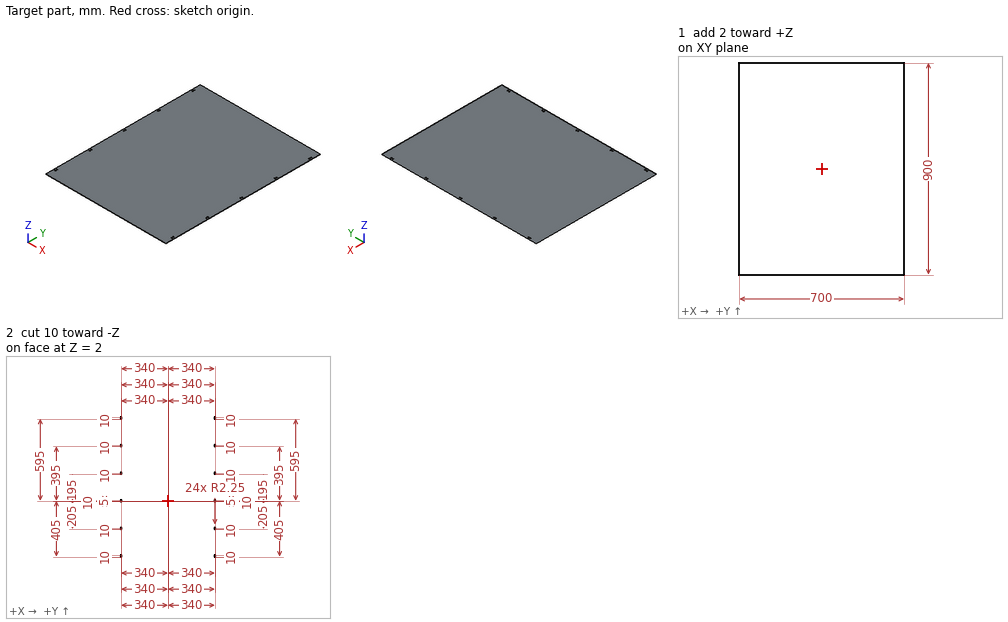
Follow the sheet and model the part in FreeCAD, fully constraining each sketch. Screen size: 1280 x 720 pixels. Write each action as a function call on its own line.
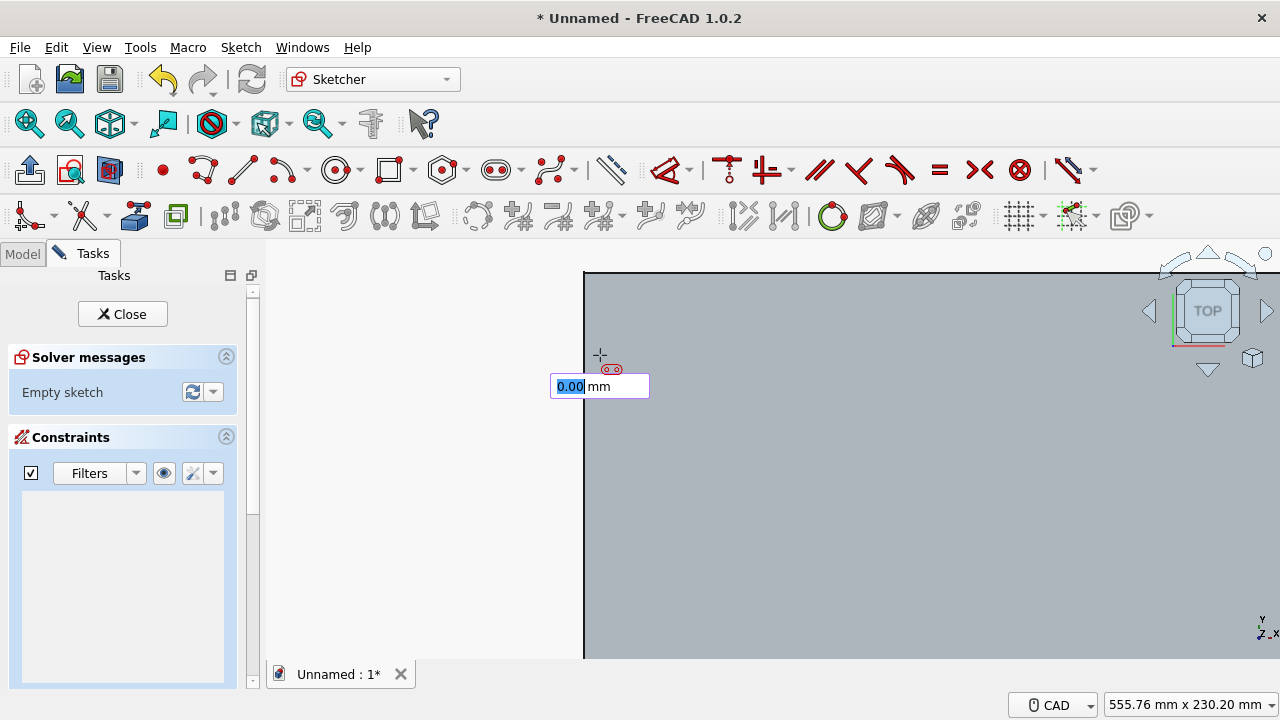
scroll(606, 364, up, 7)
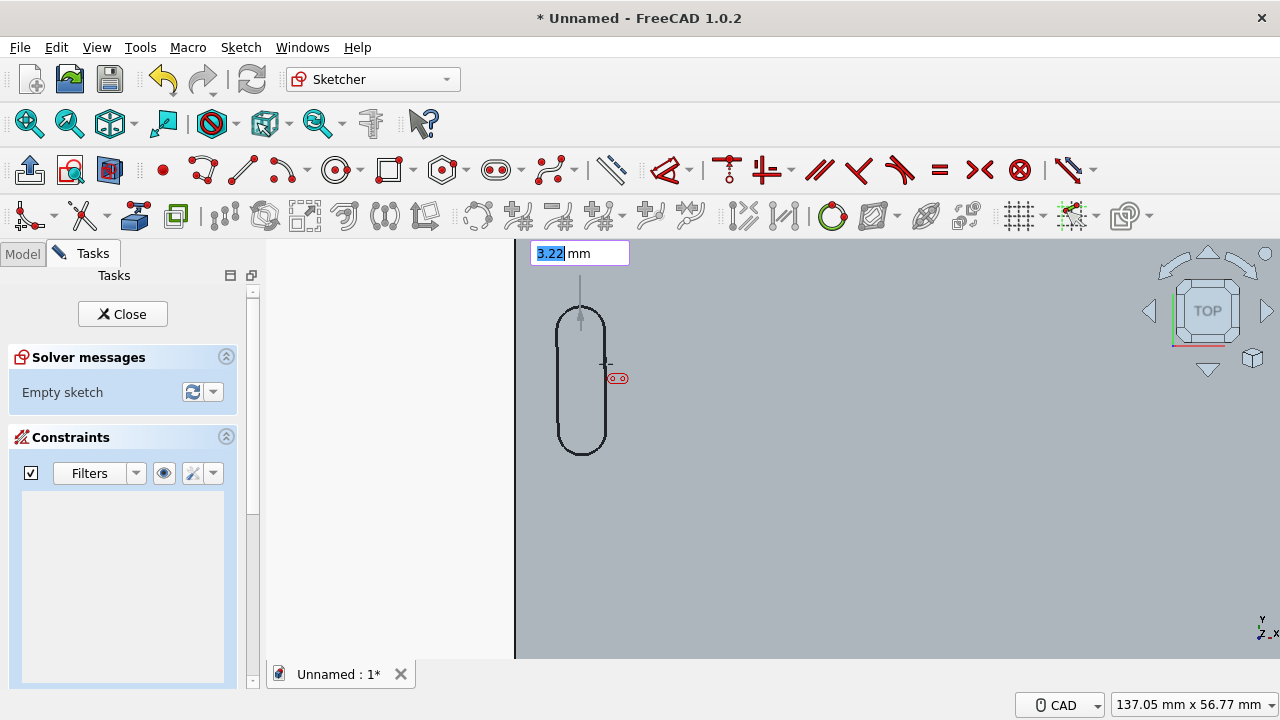
click(606, 362)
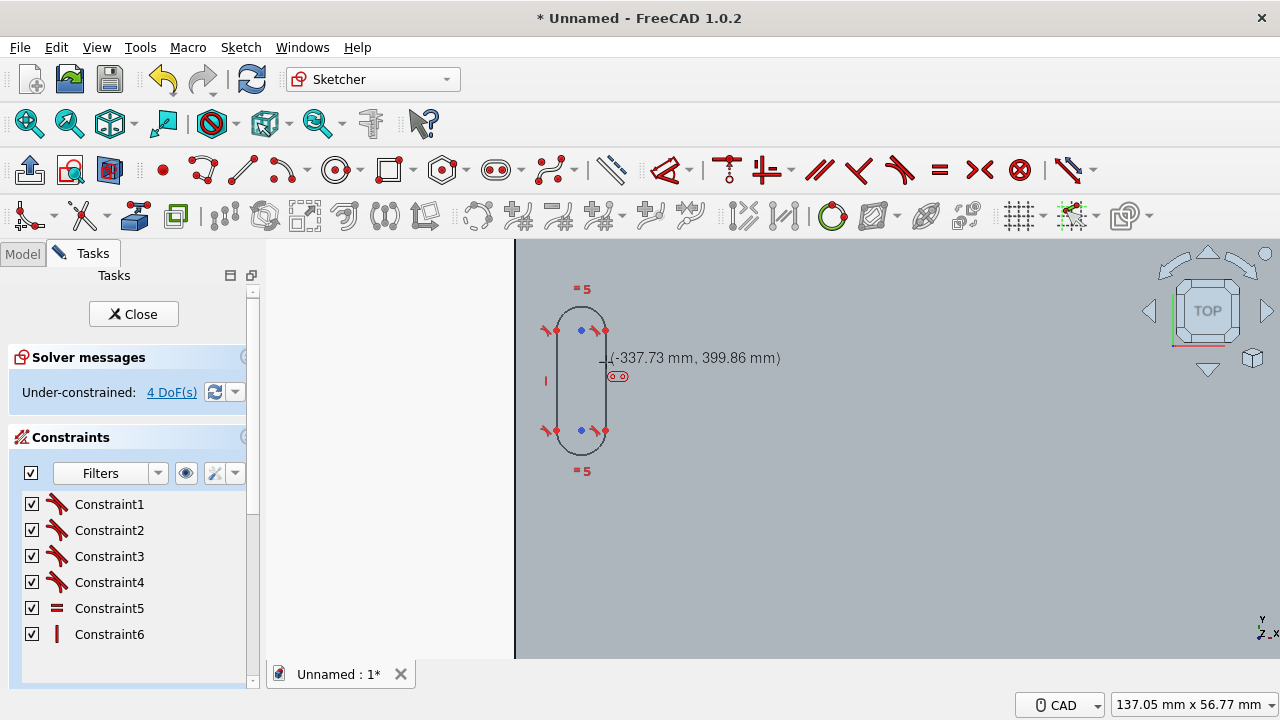
scroll(603, 358, down, 16)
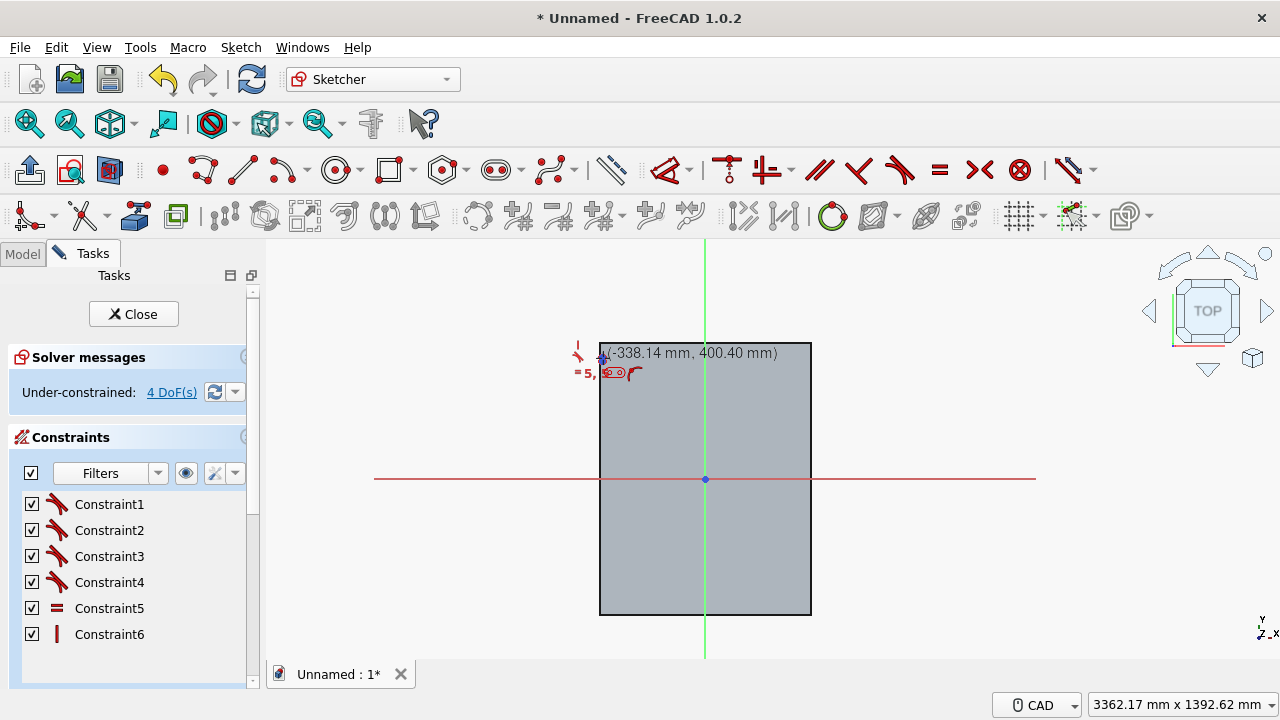
scroll(808, 360, up, 18)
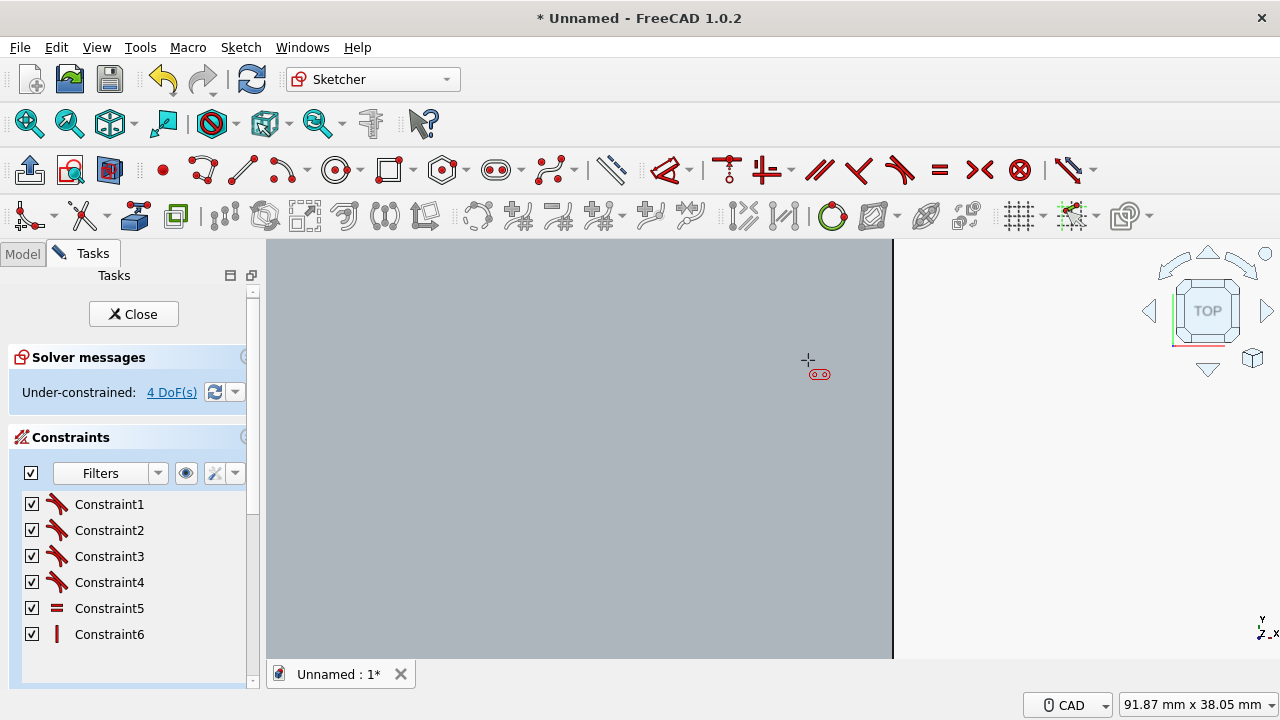
scroll(808, 360, down, 18)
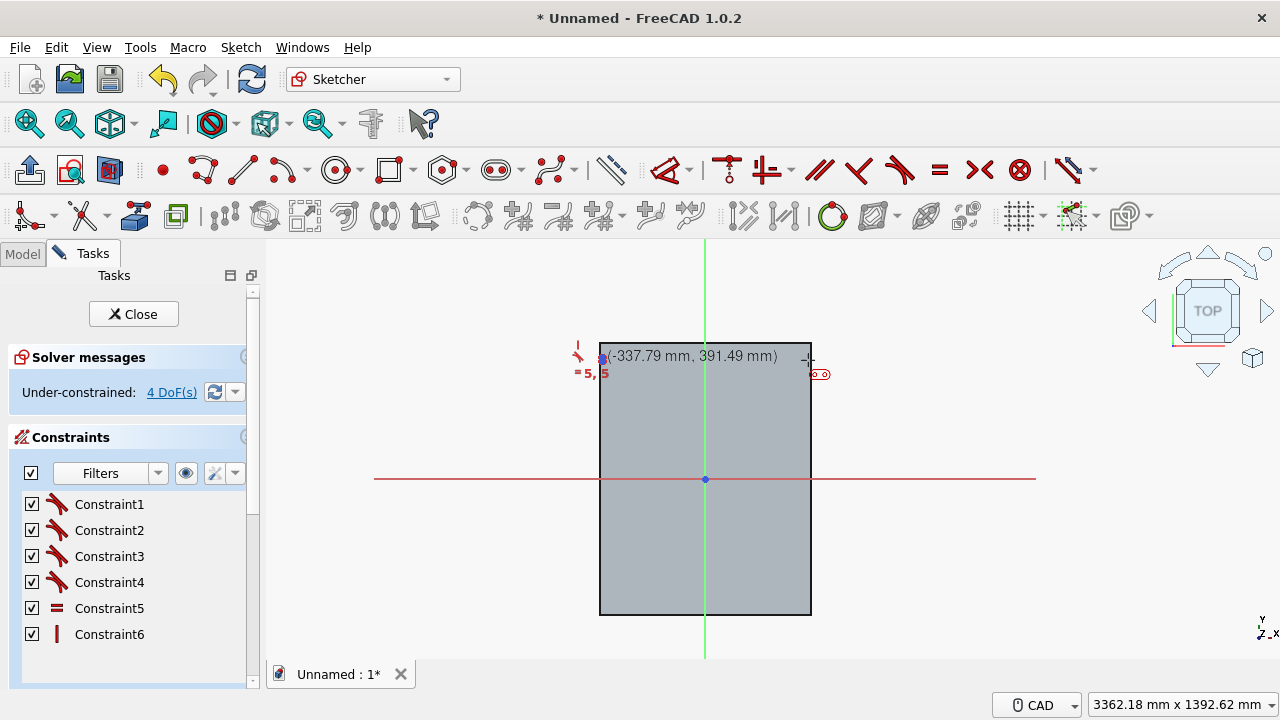
click(808, 360)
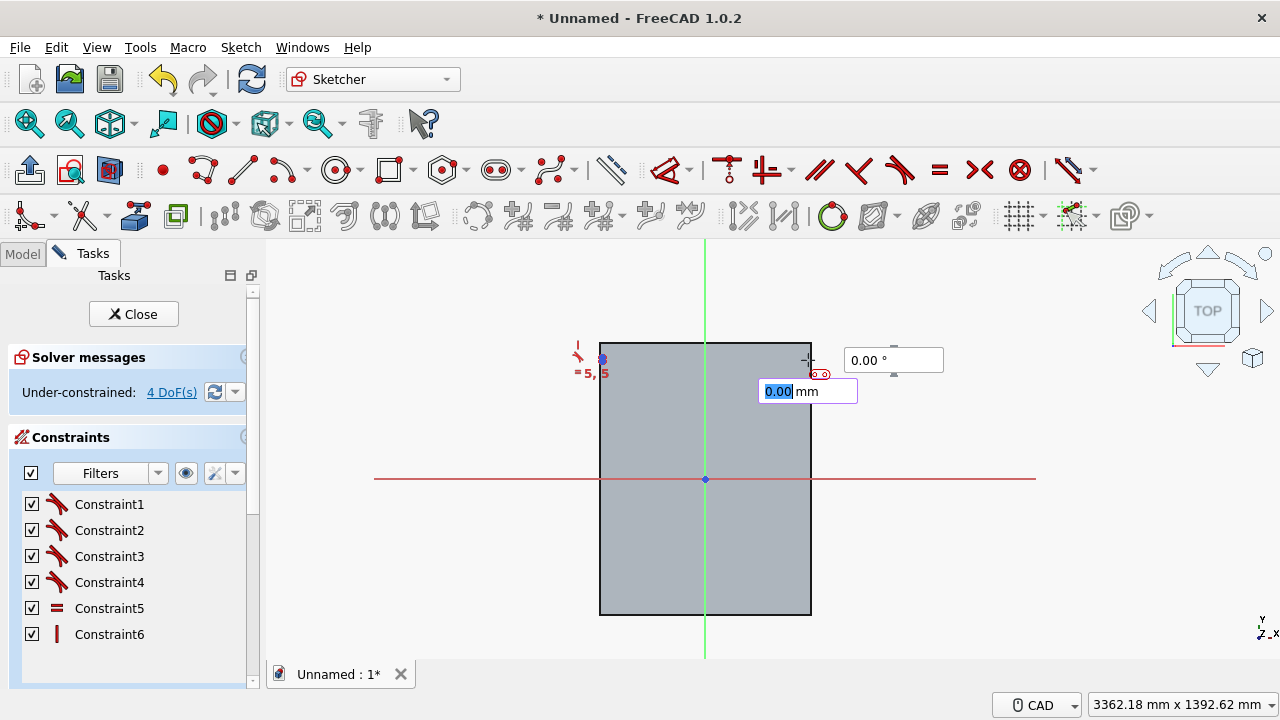
scroll(808, 357, up, 9)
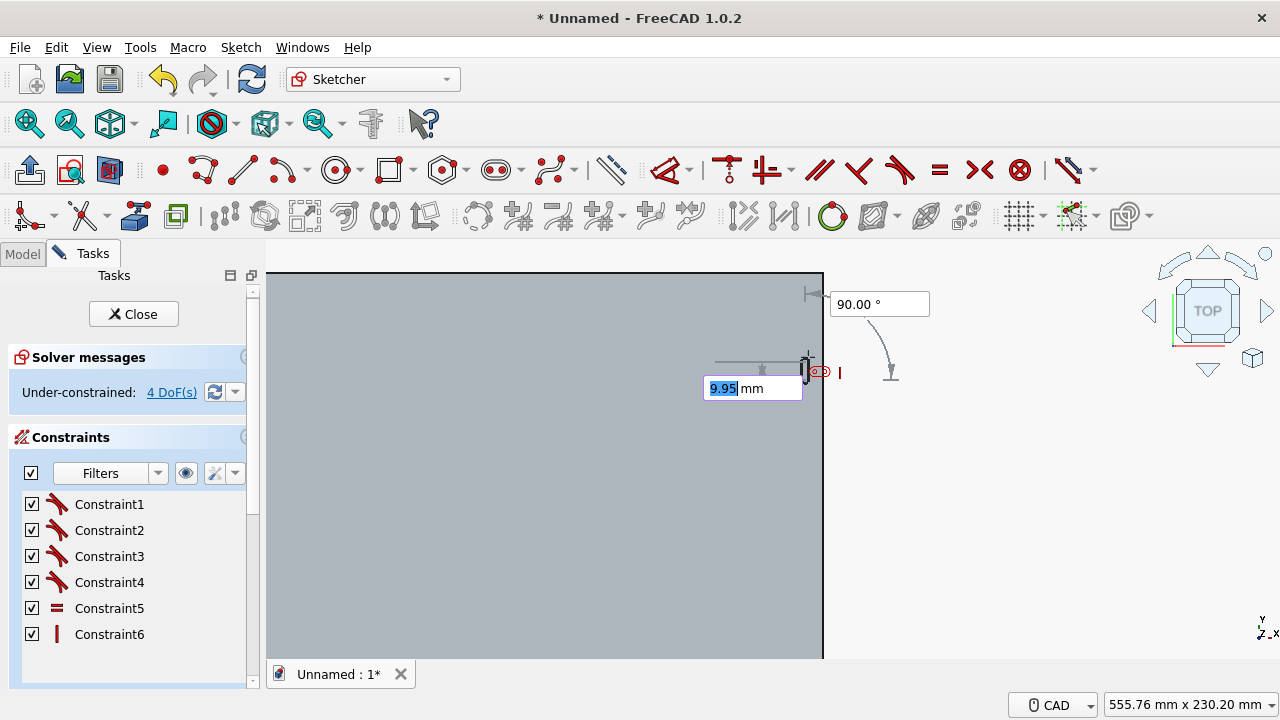
click(805, 355)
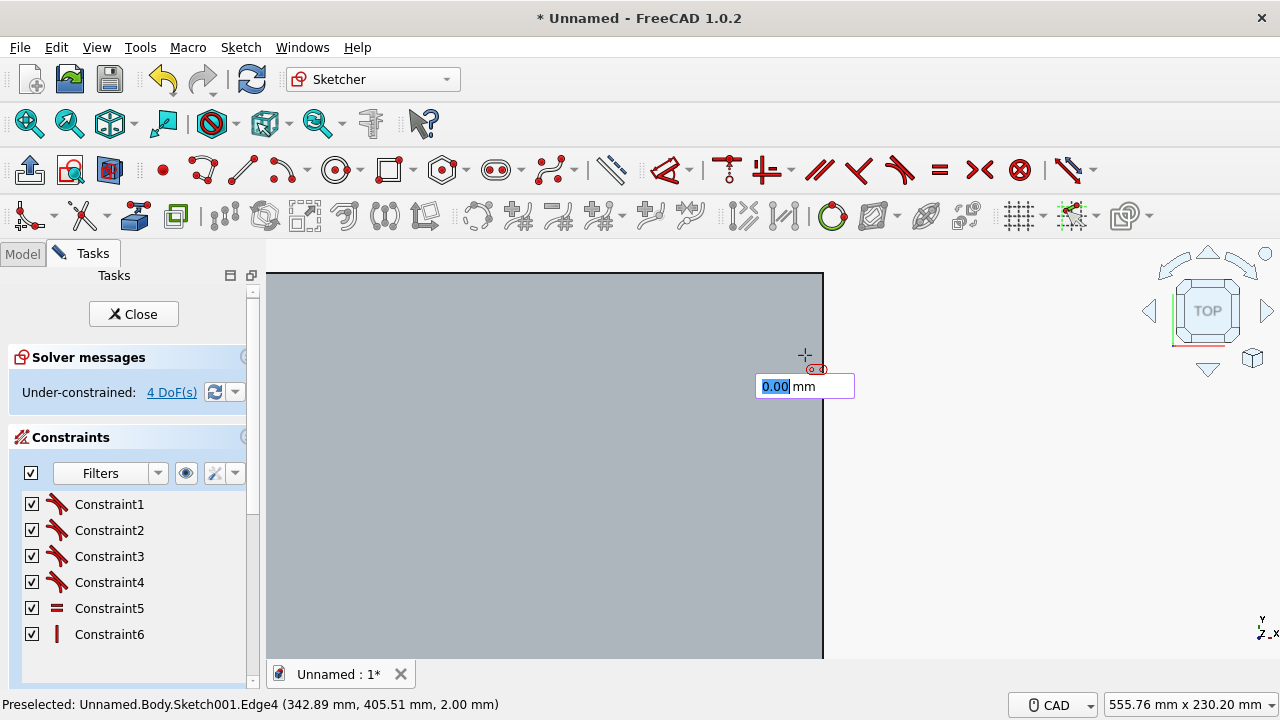
scroll(800, 364, up, 7)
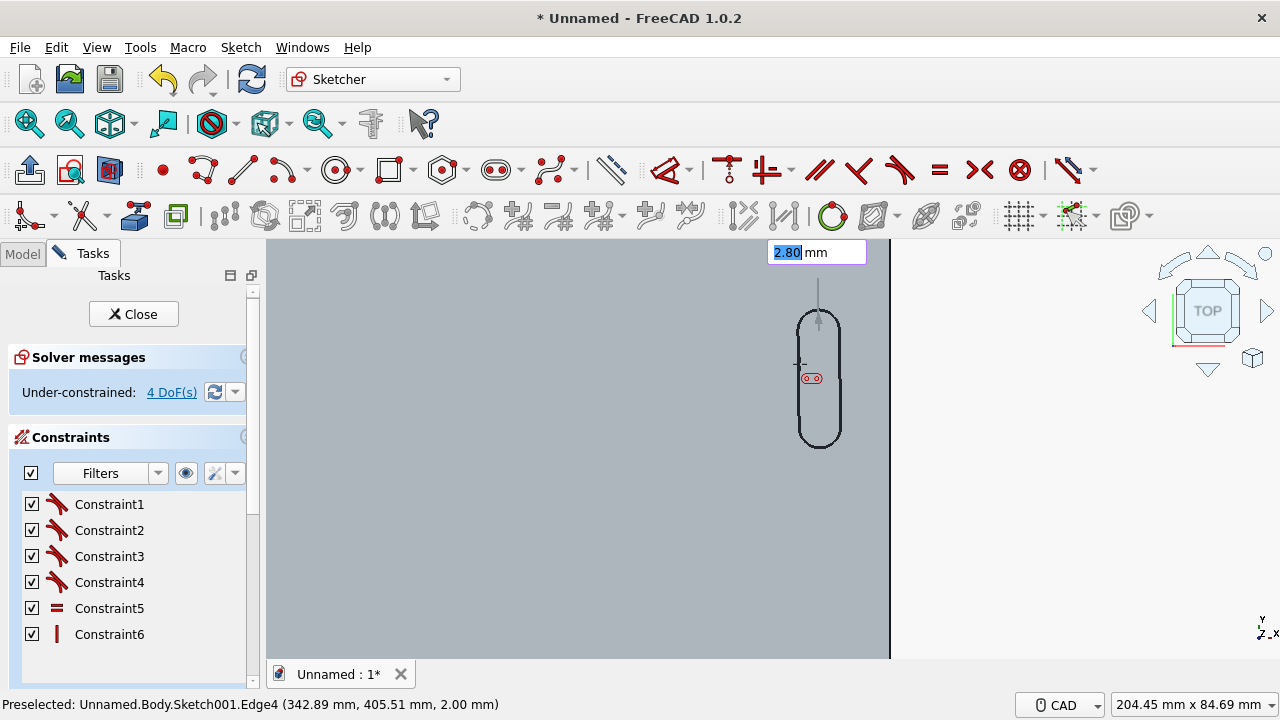
click(799, 364)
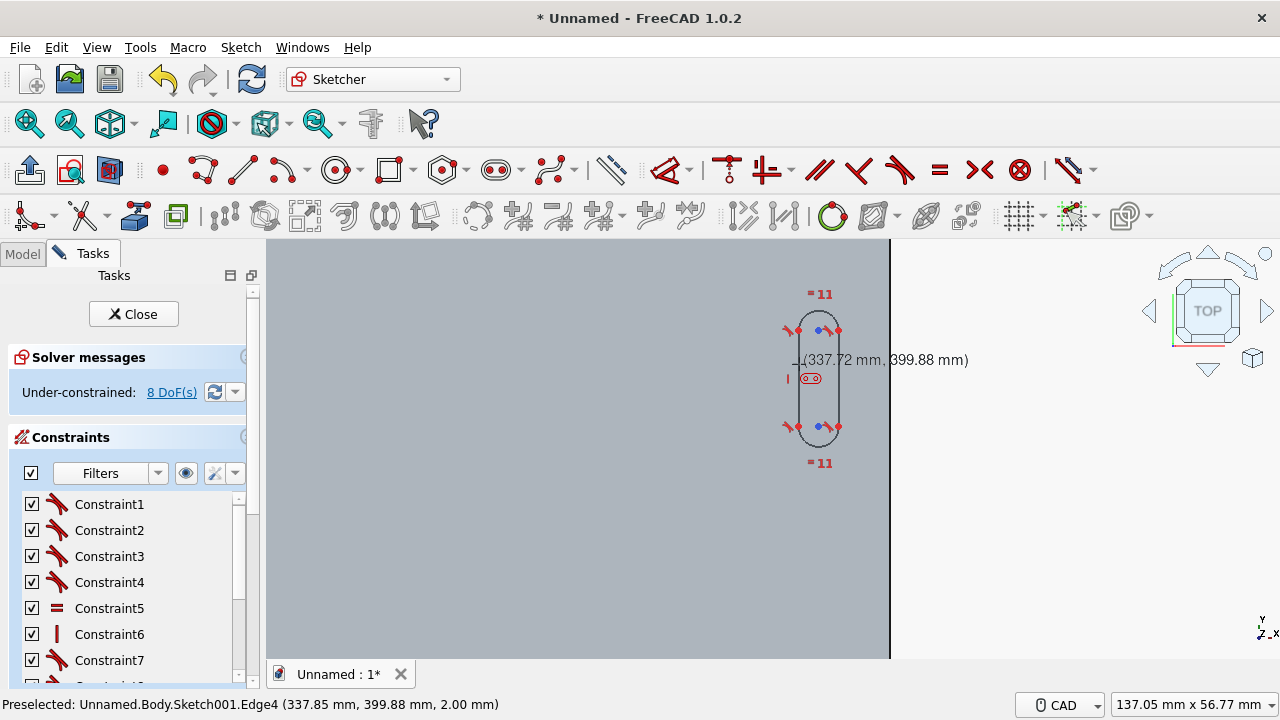
scroll(807, 358, down, 16)